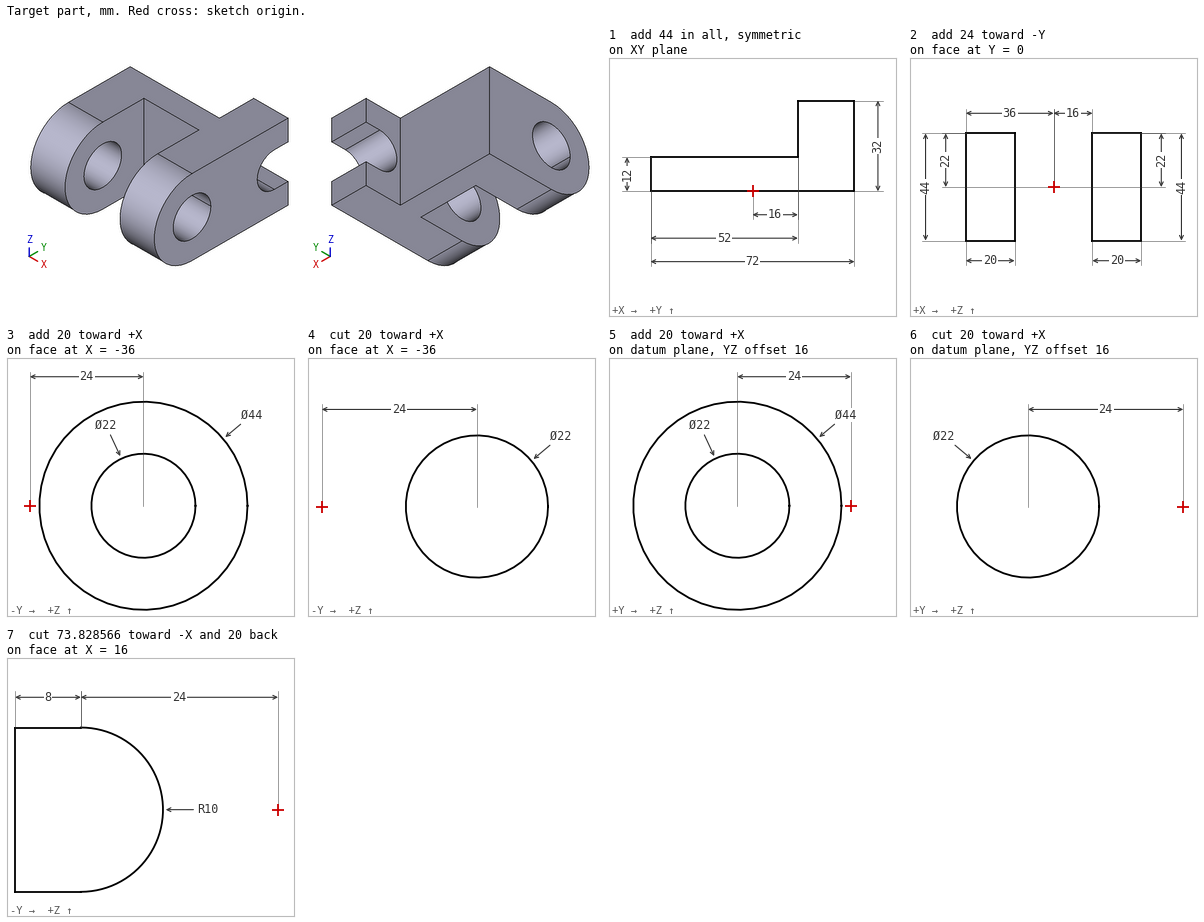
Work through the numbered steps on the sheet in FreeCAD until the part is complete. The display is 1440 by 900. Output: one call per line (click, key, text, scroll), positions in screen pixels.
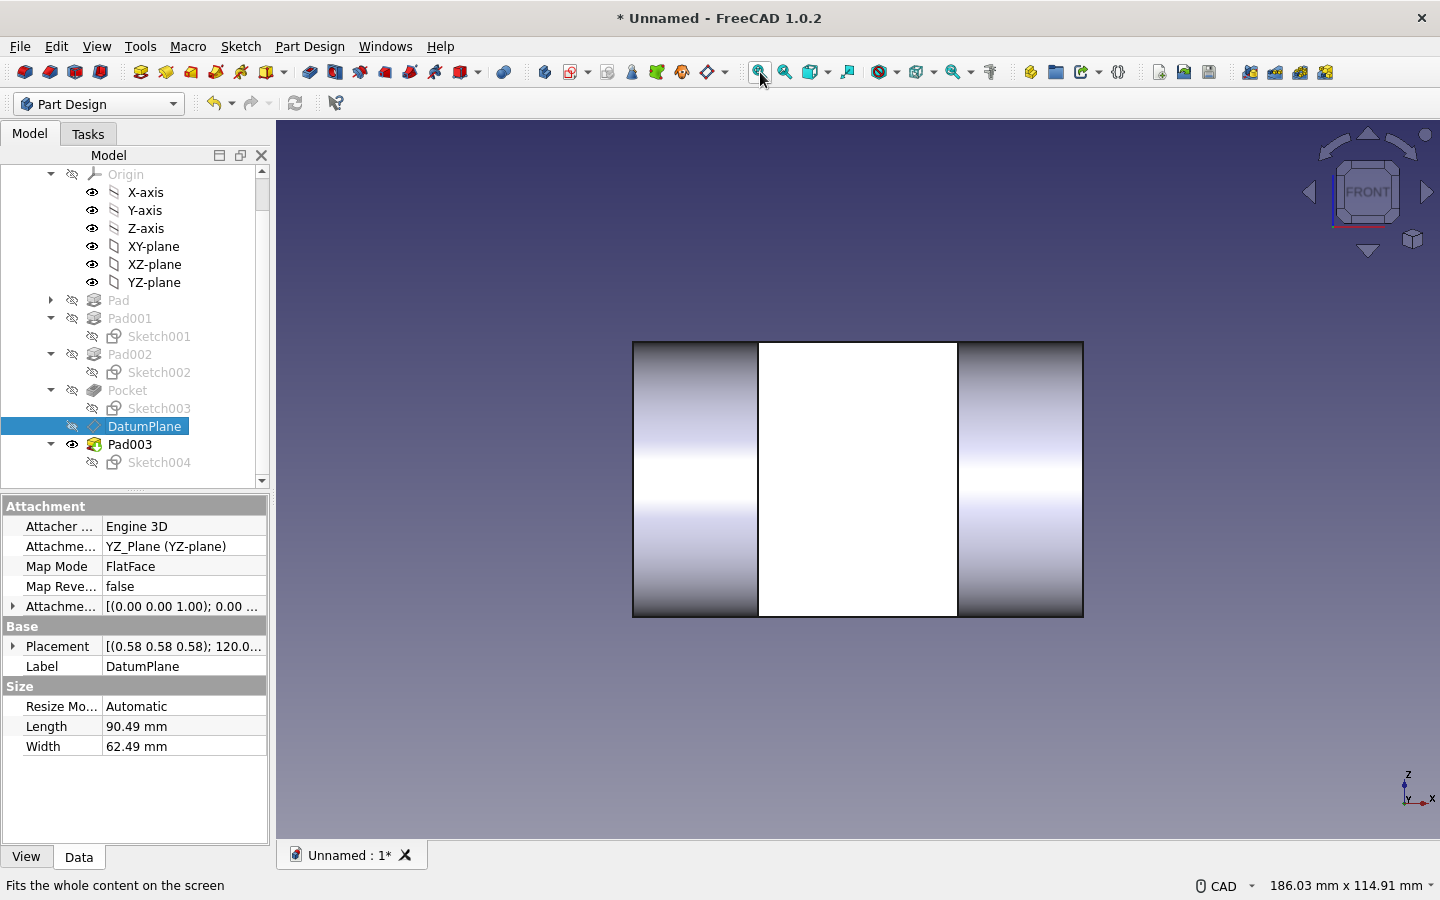
click(137, 282)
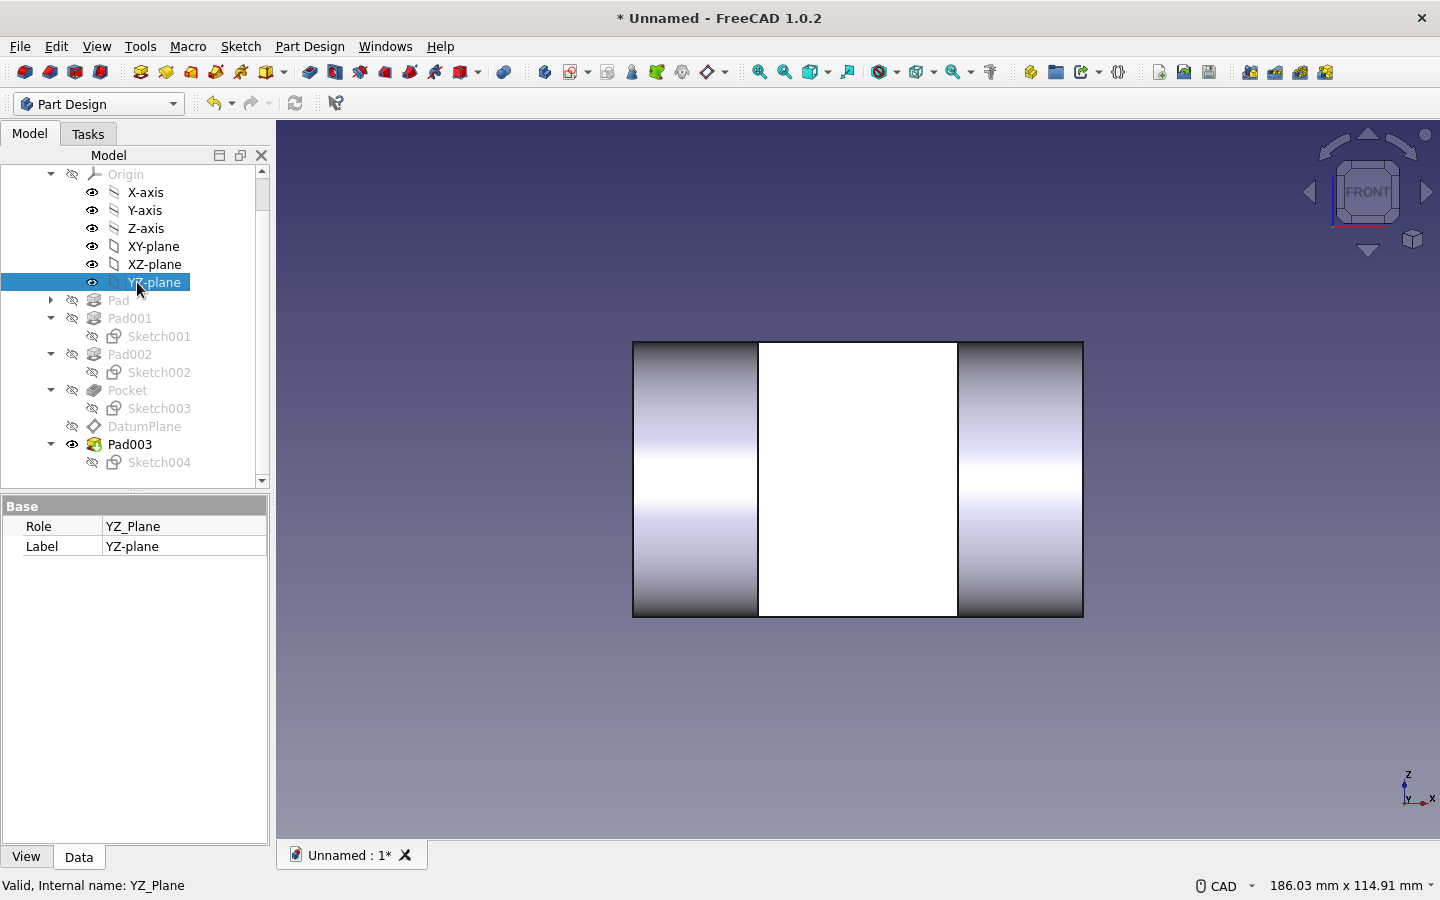
click(706, 72)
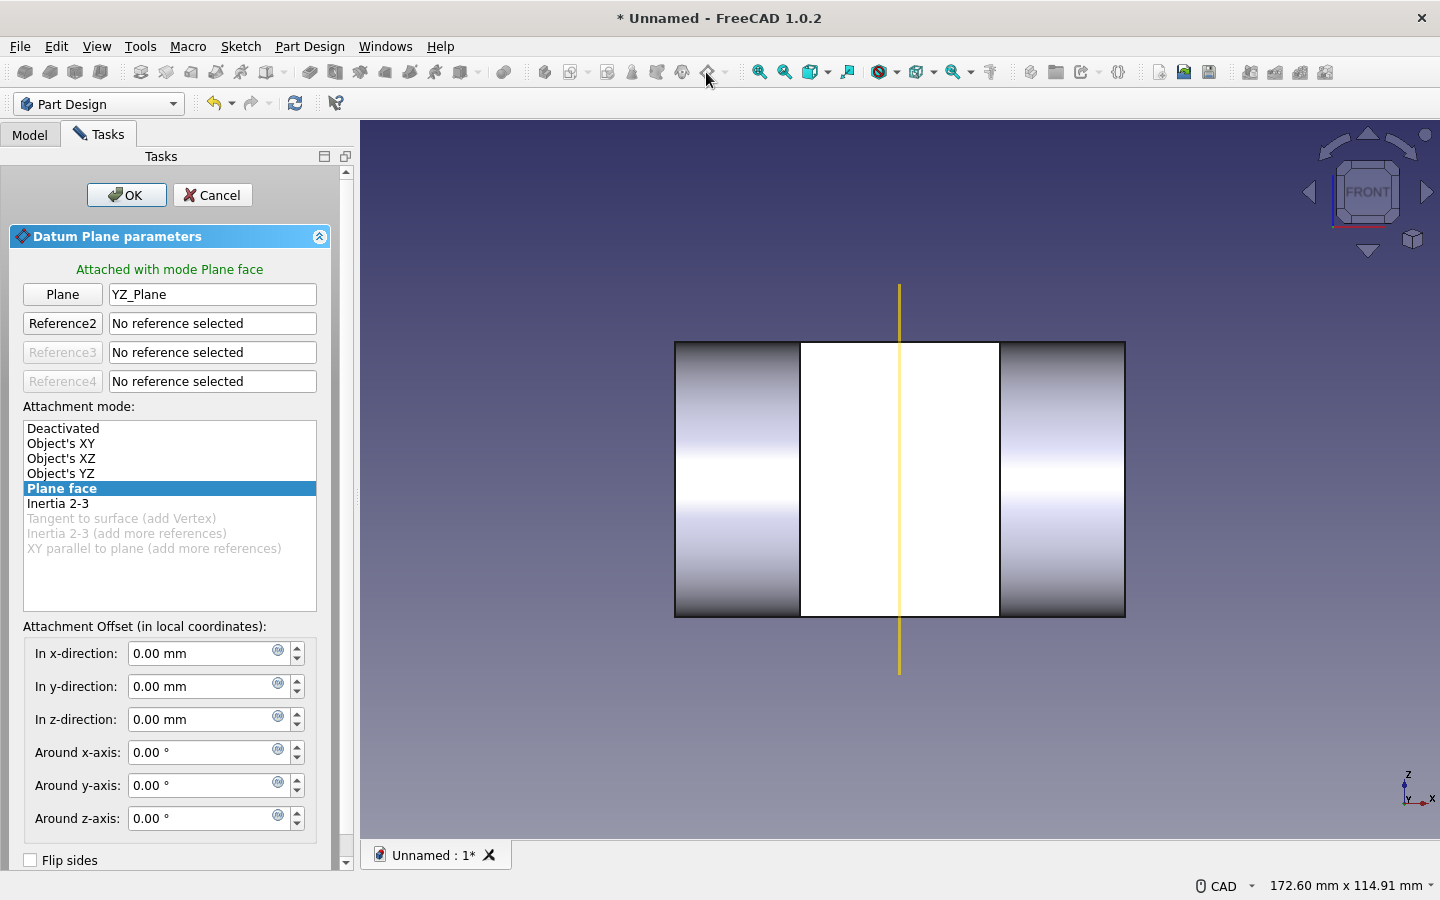
triple_click(210, 720)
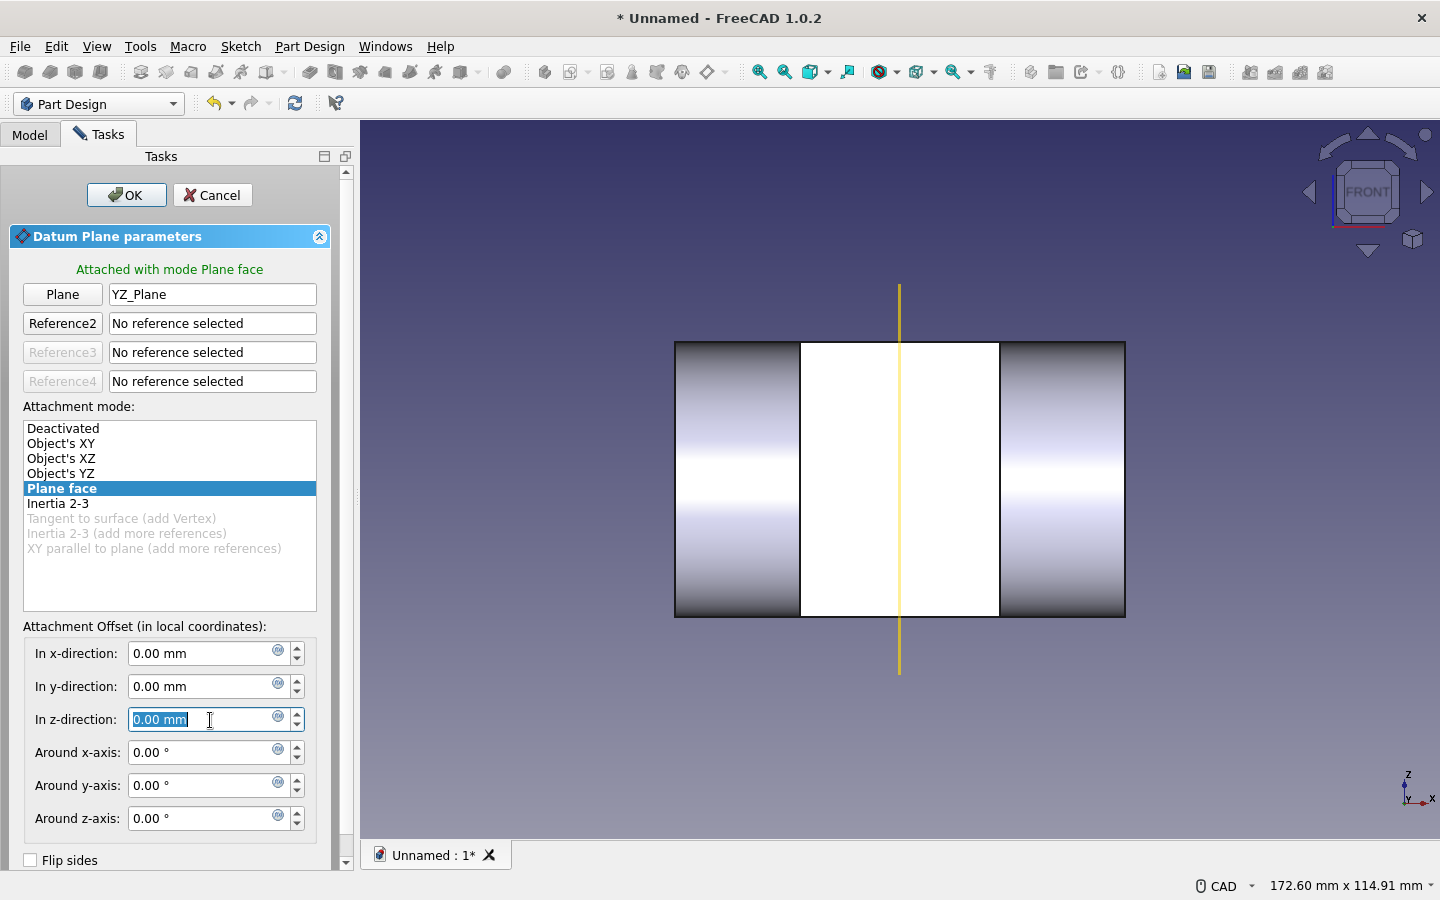
text(16)
key(Tab)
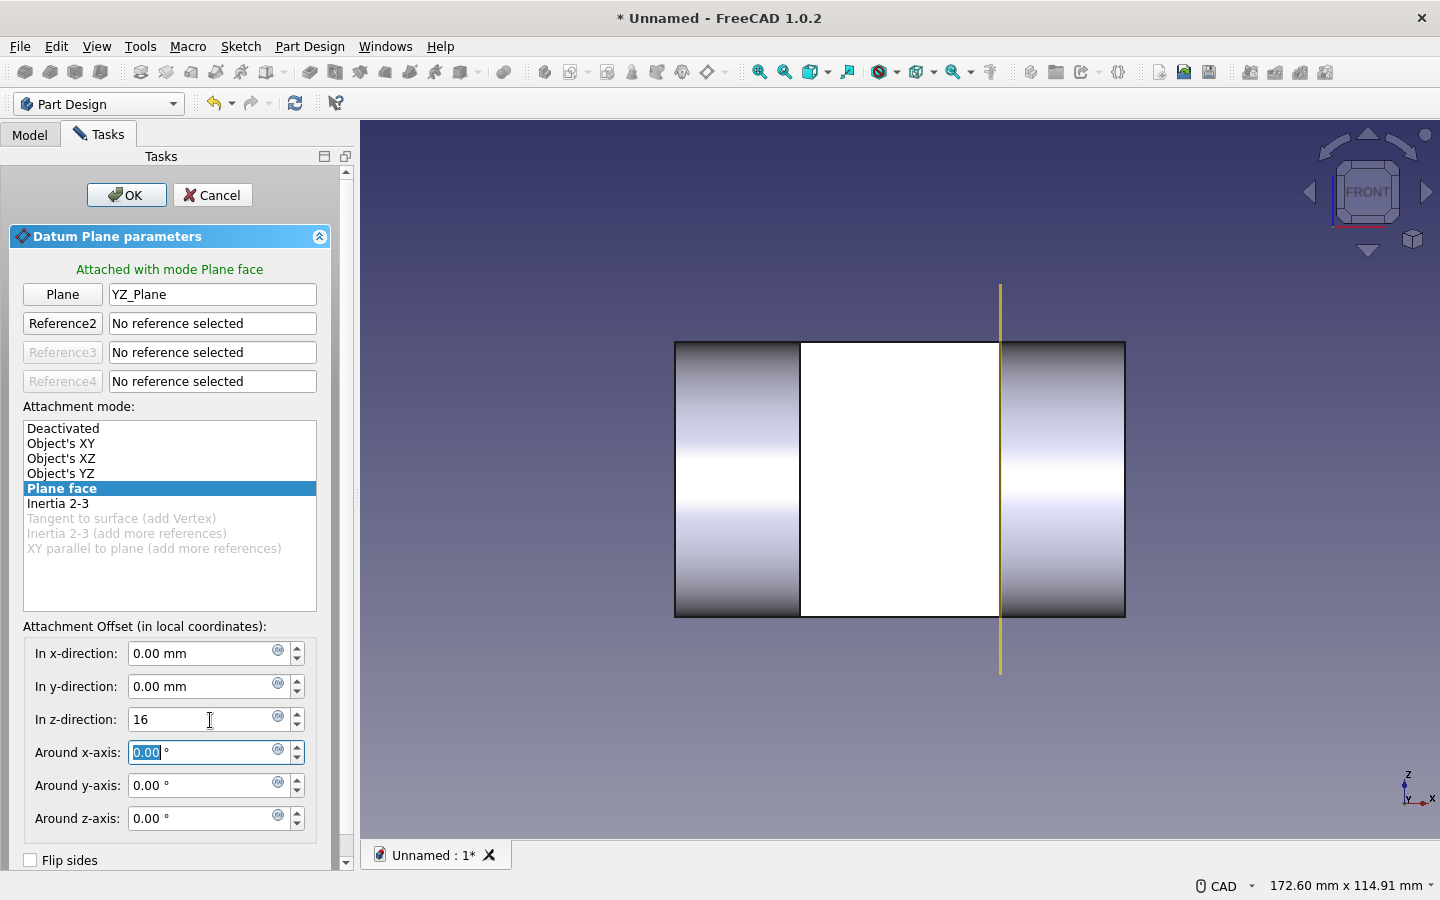
click(127, 195)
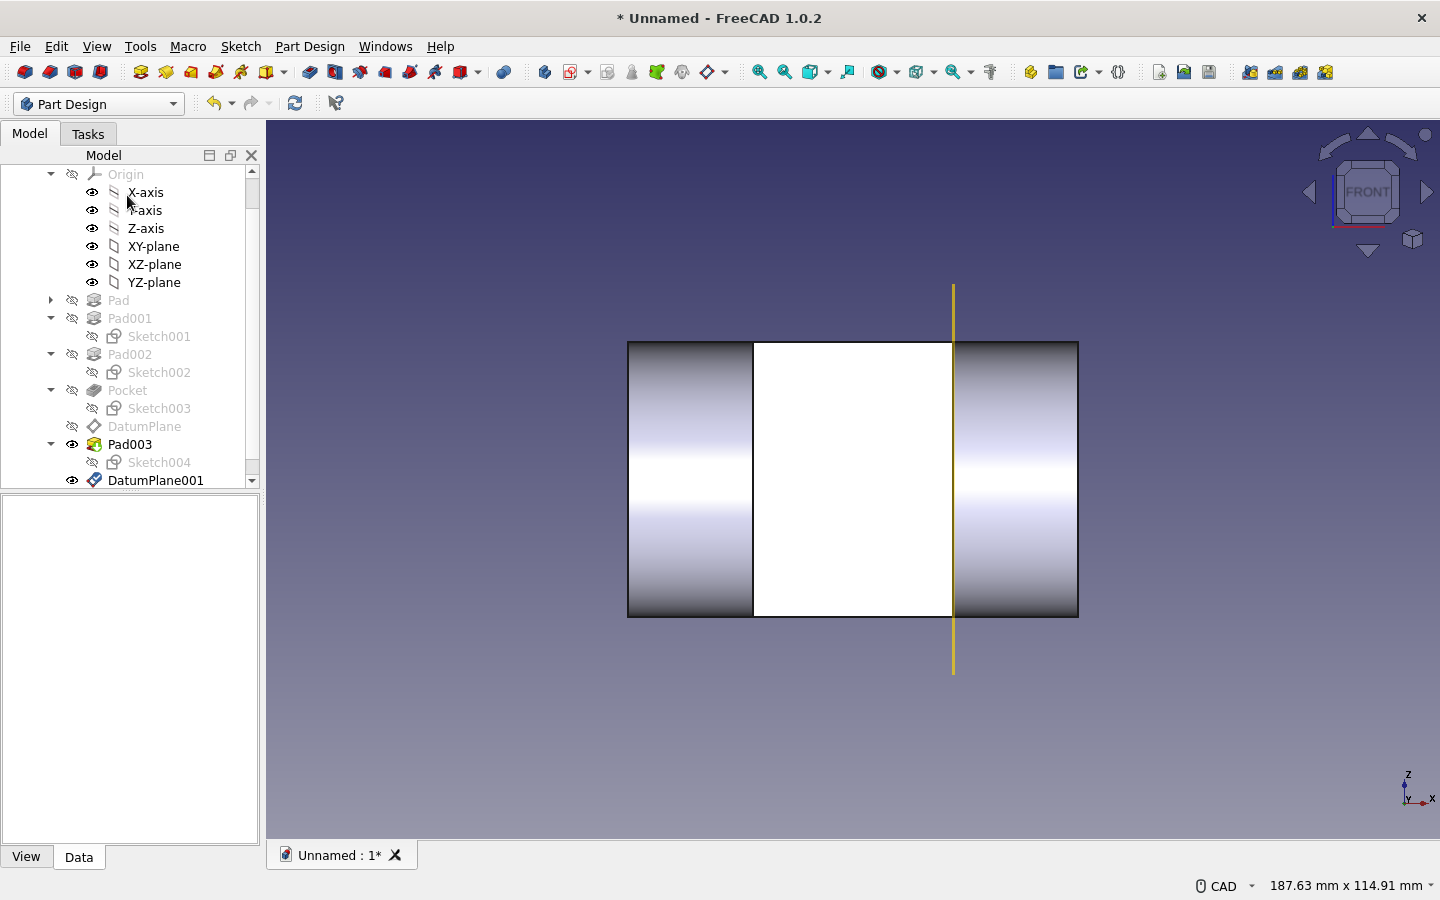
click(117, 480)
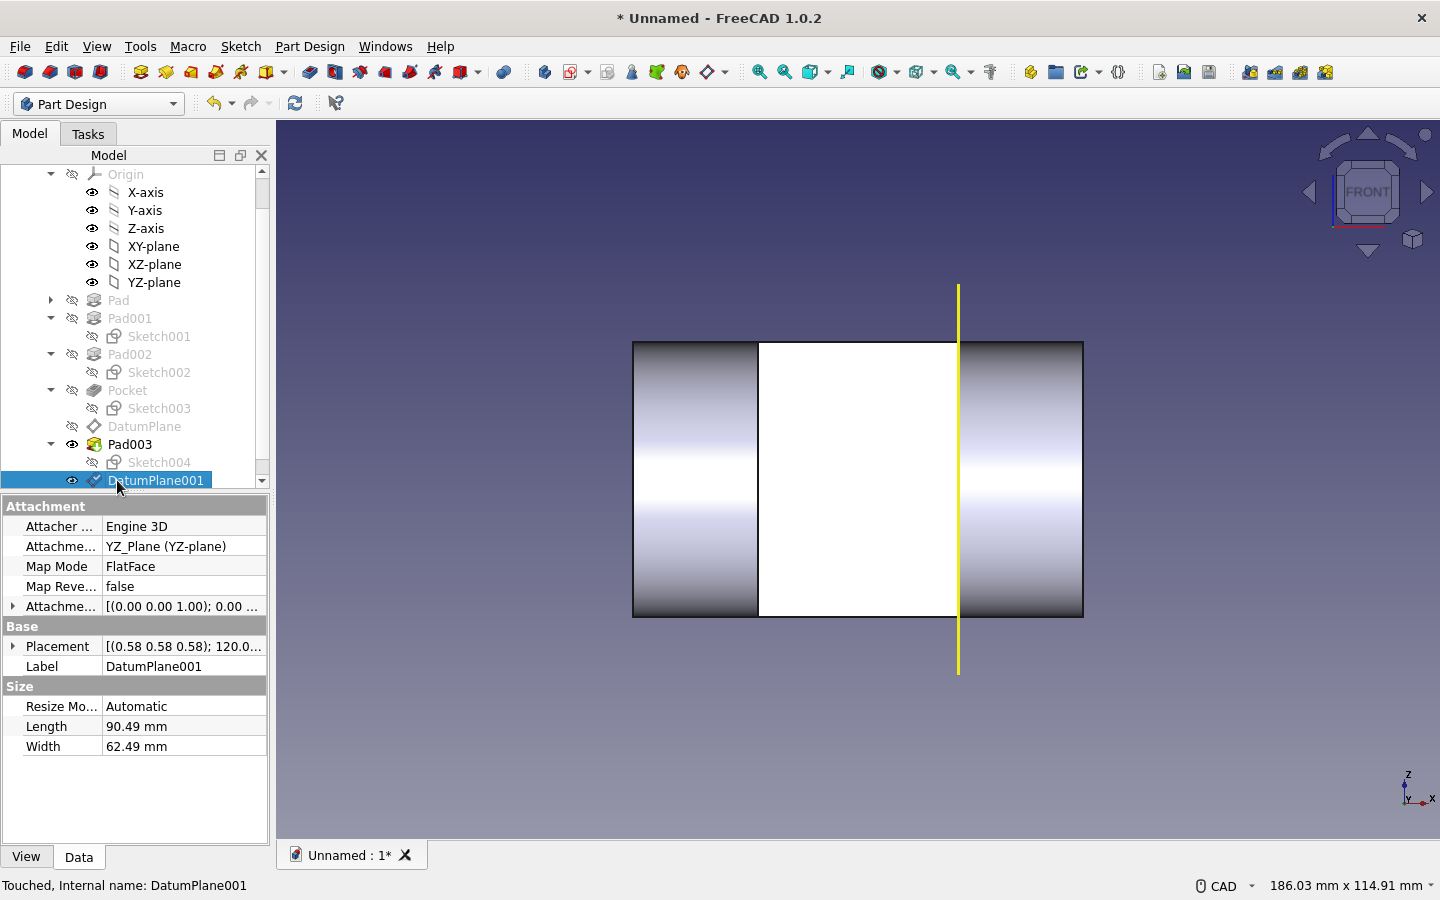
click(570, 72)